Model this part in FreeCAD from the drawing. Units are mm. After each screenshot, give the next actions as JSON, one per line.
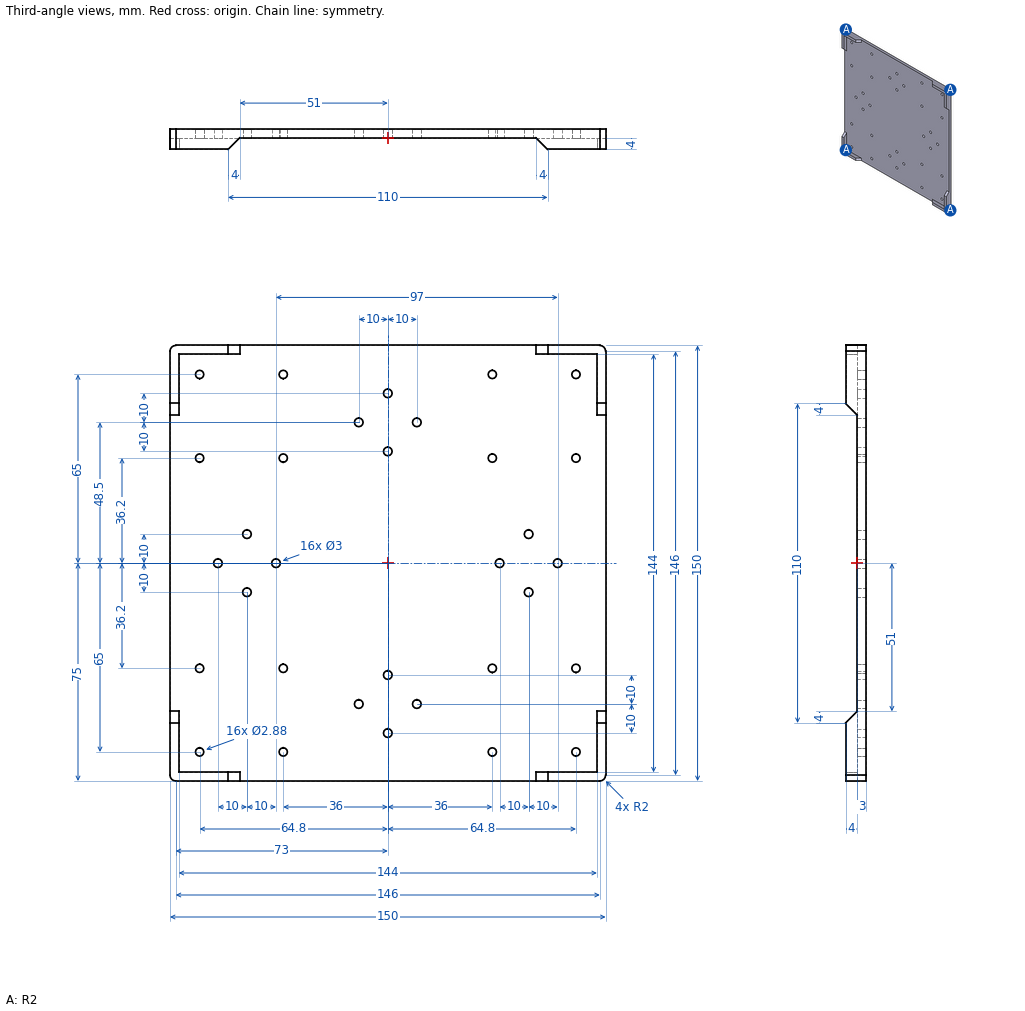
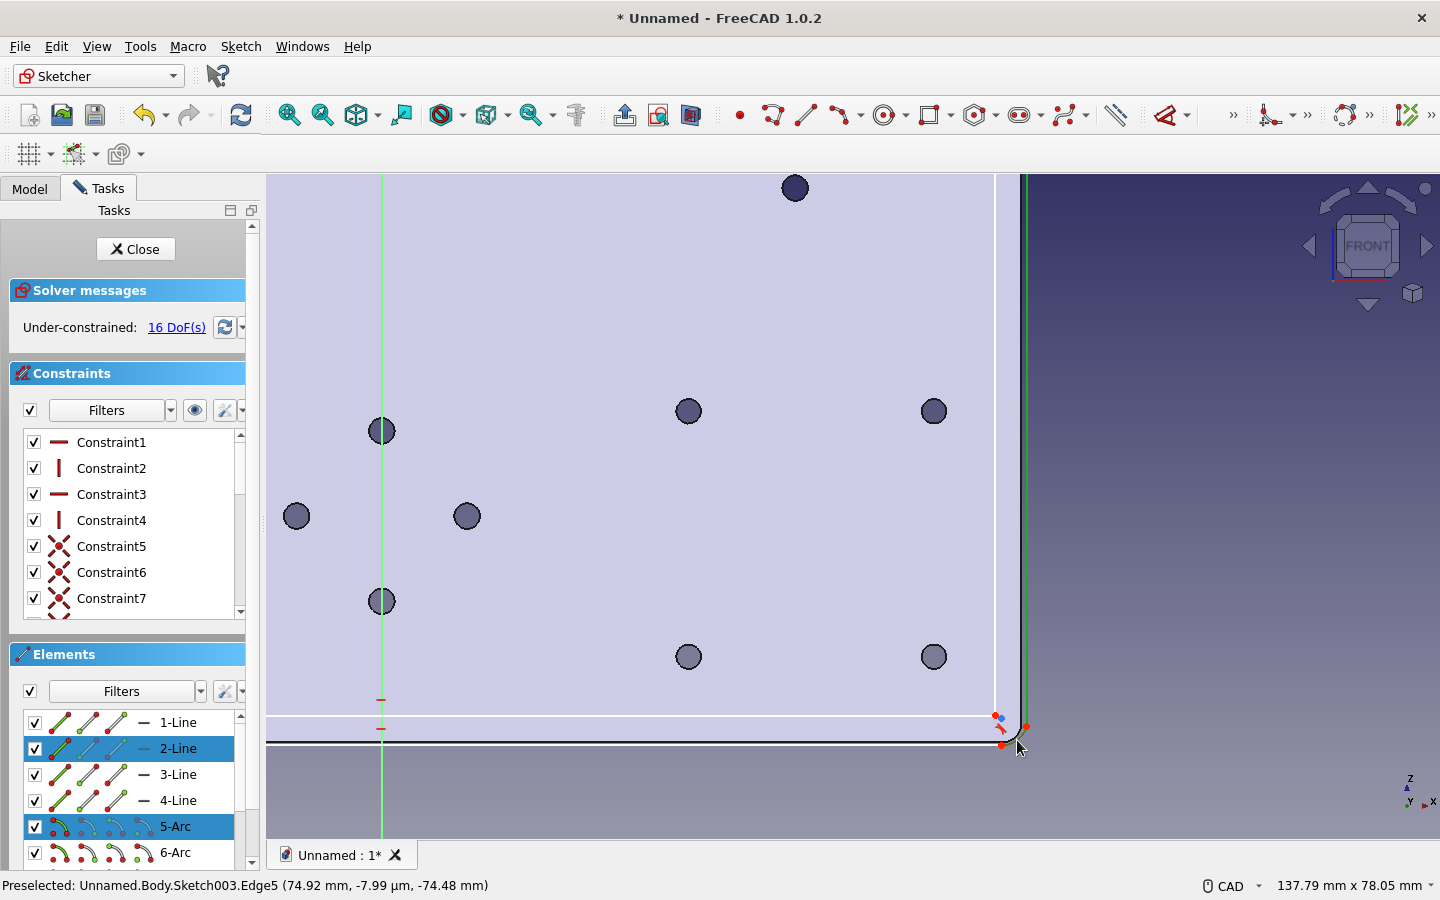
{"action": "key", "text": "t"}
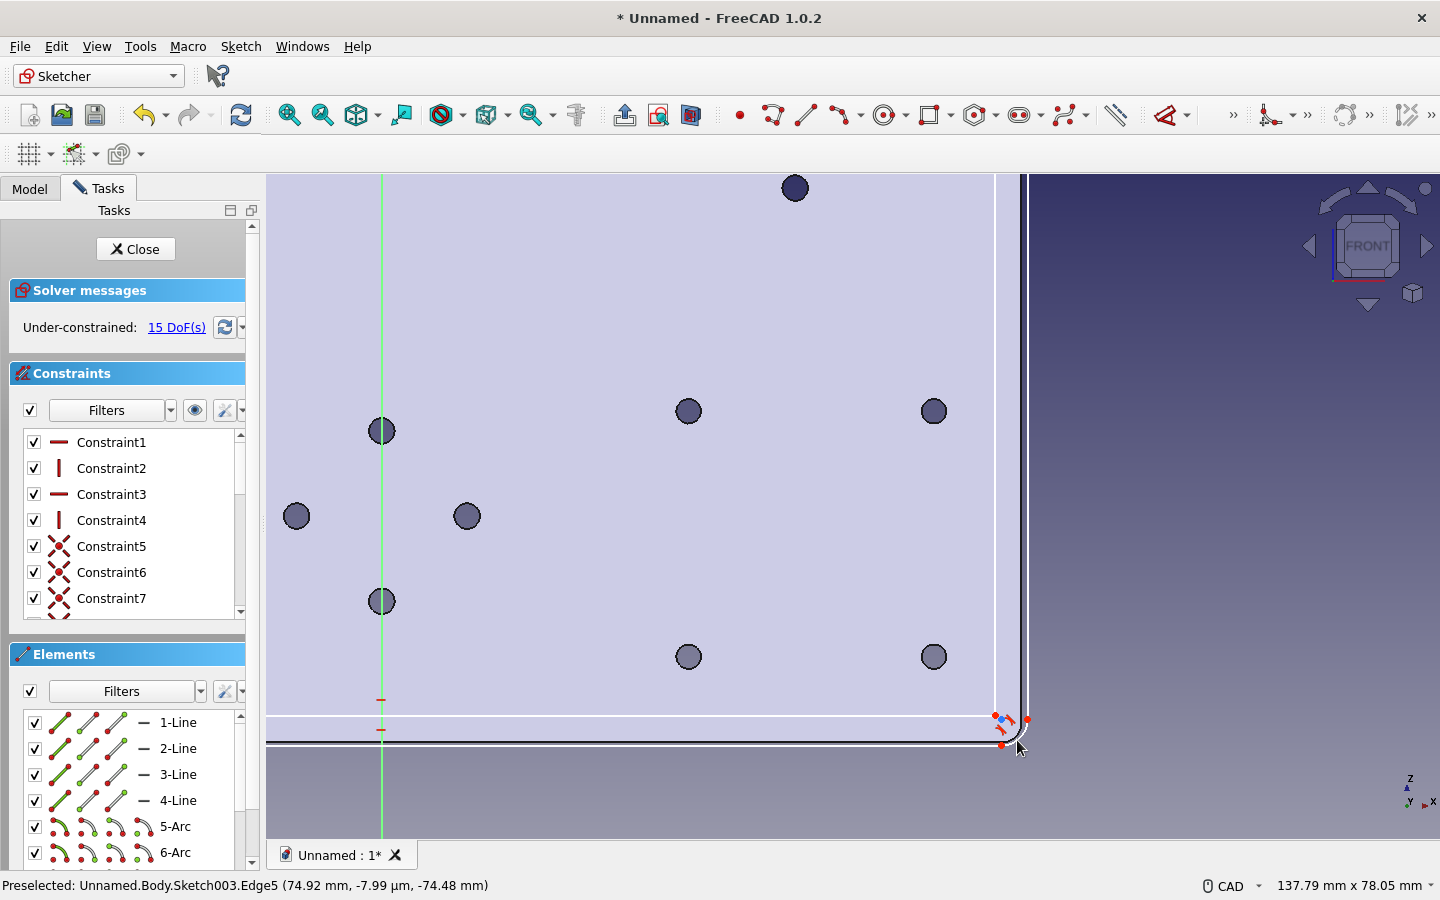
{"action": "left_click", "coordinate": [1028, 349]}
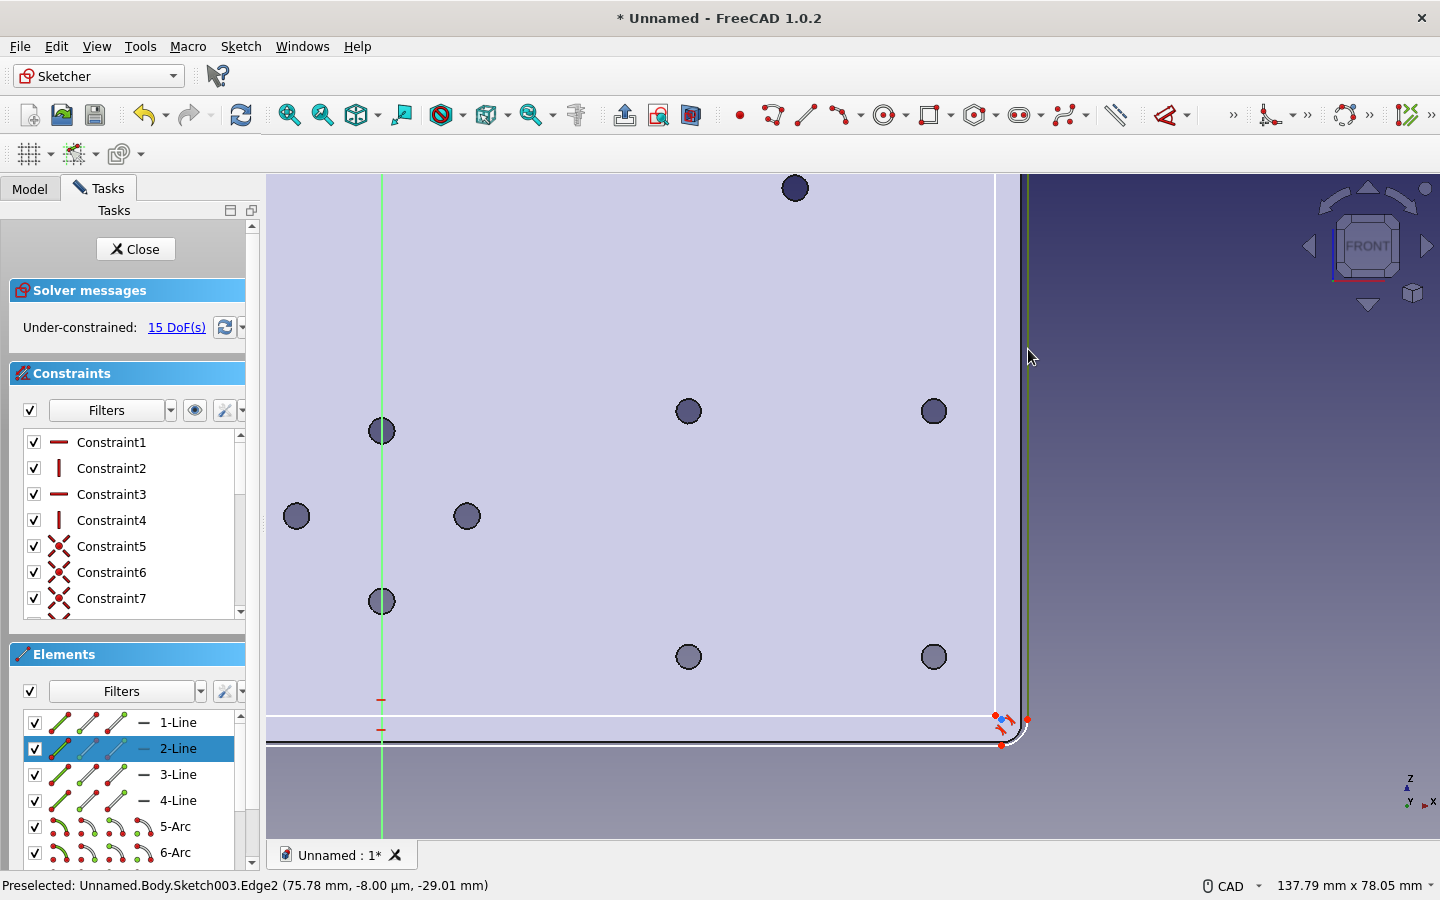
{"action": "scroll", "coordinate": [1019, 741], "scroll_direction": "down", "scroll_amount": 5}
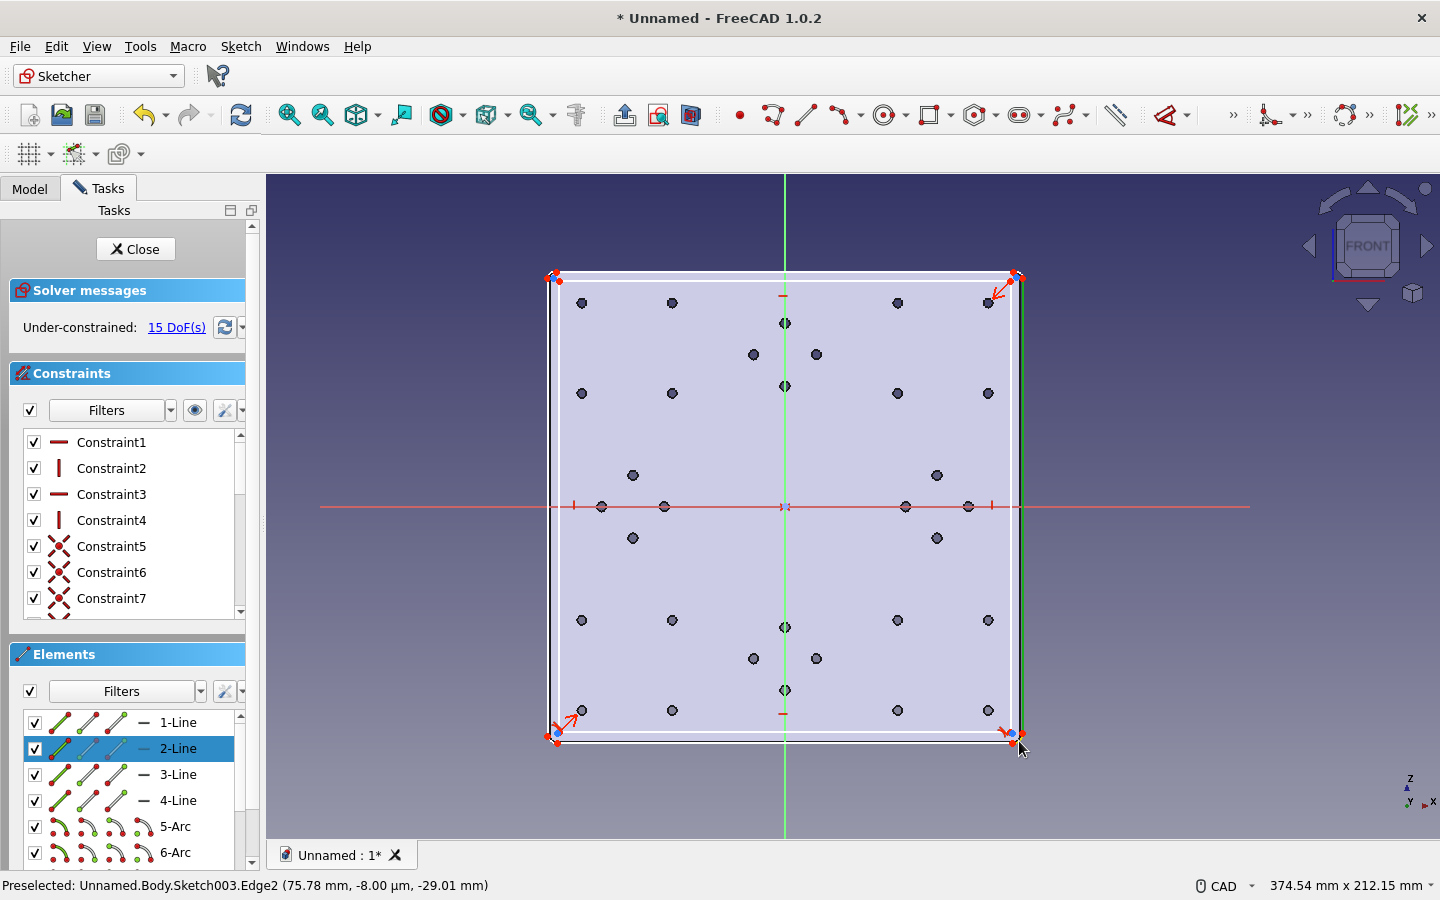
{"action": "scroll", "coordinate": [1022, 275], "scroll_direction": "up", "scroll_amount": 7}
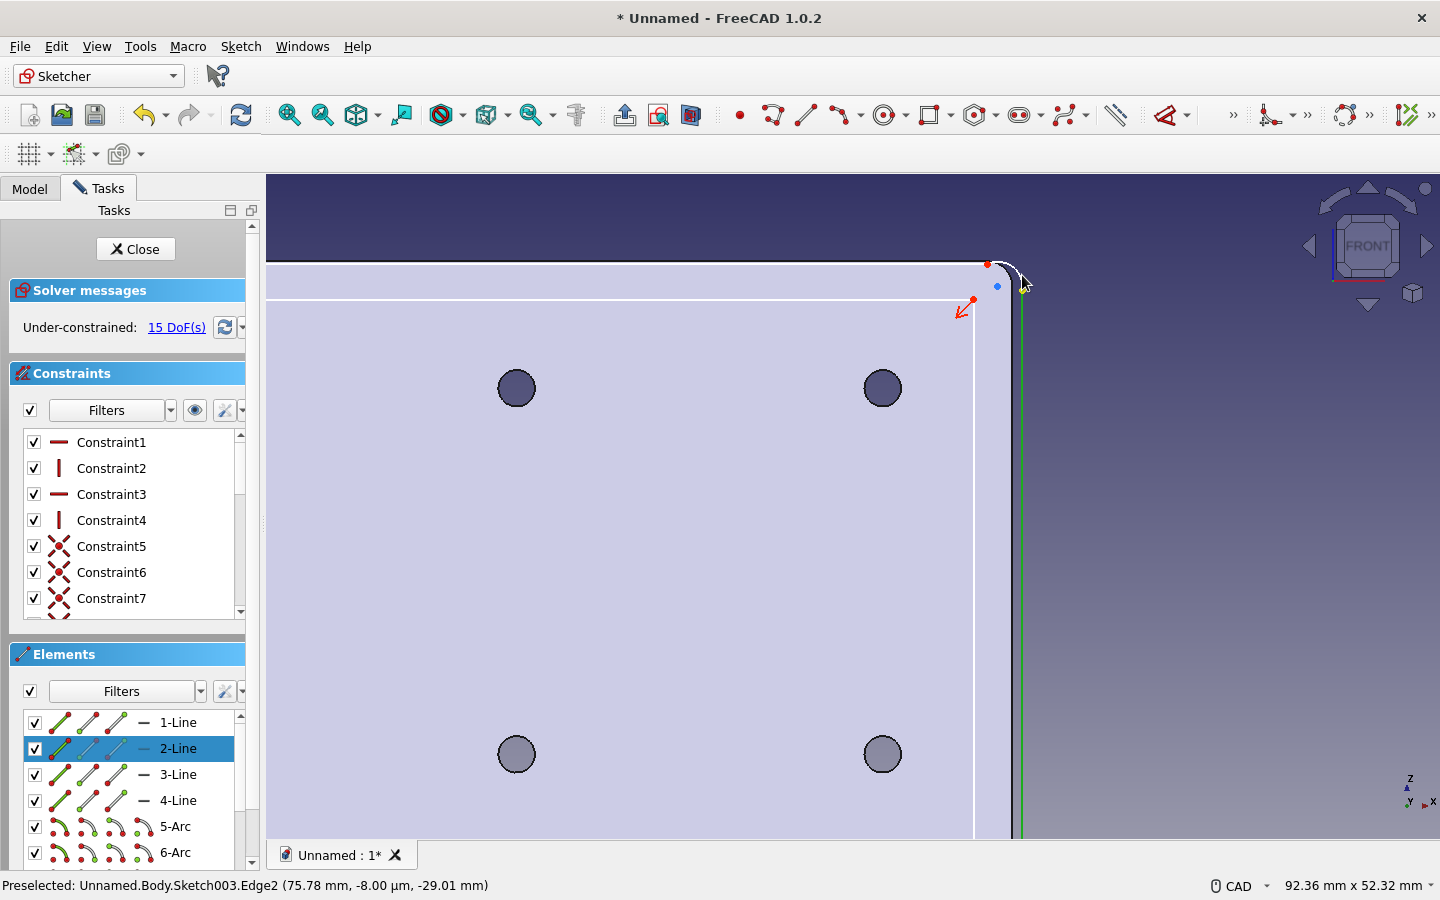
{"action": "left_click", "coordinate": [1019, 275]}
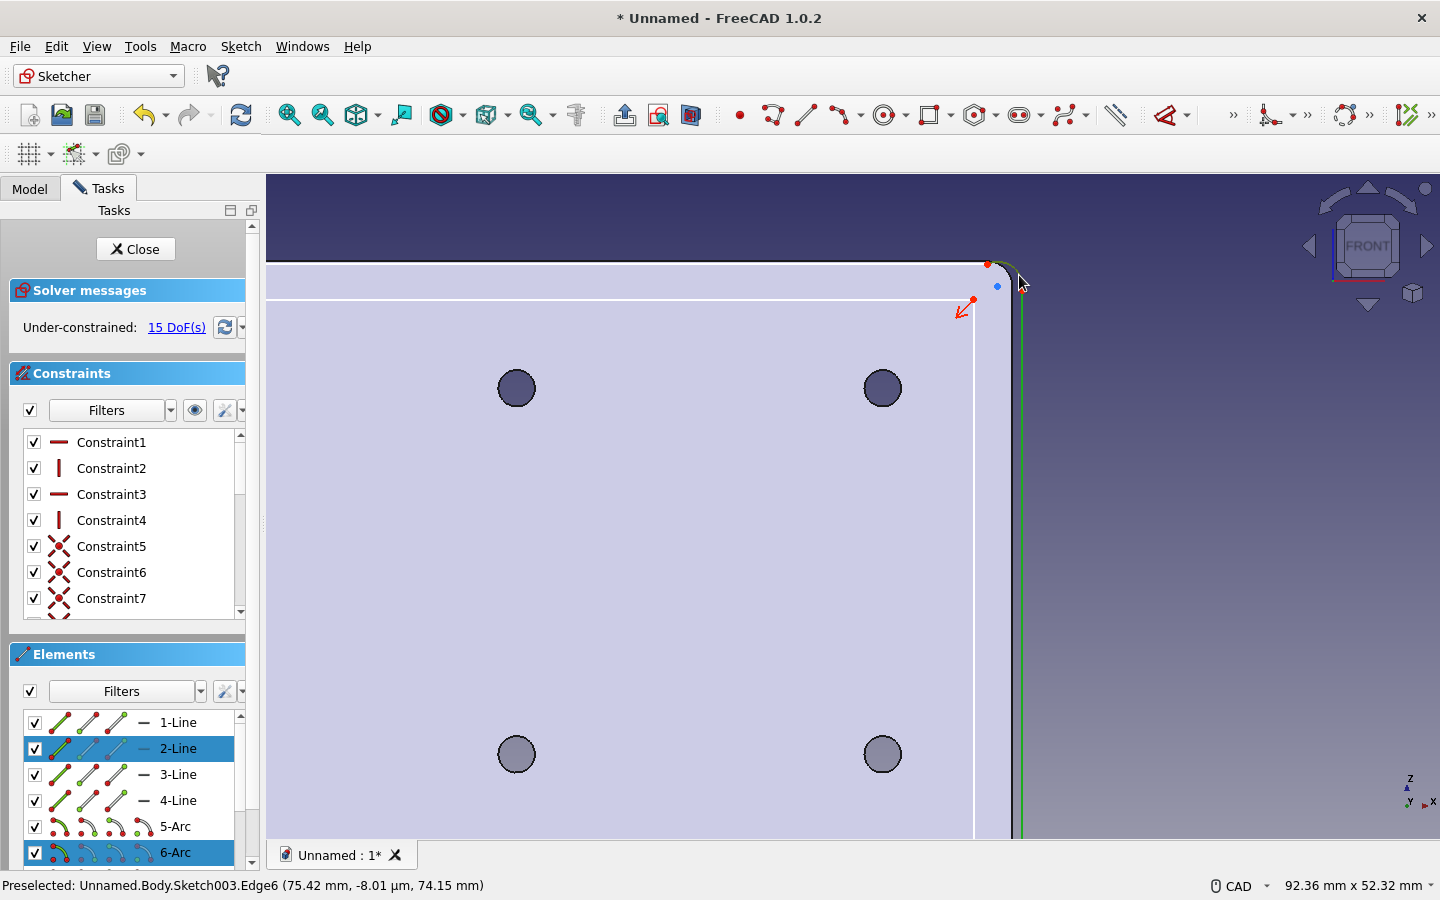
{"action": "key", "text": "t"}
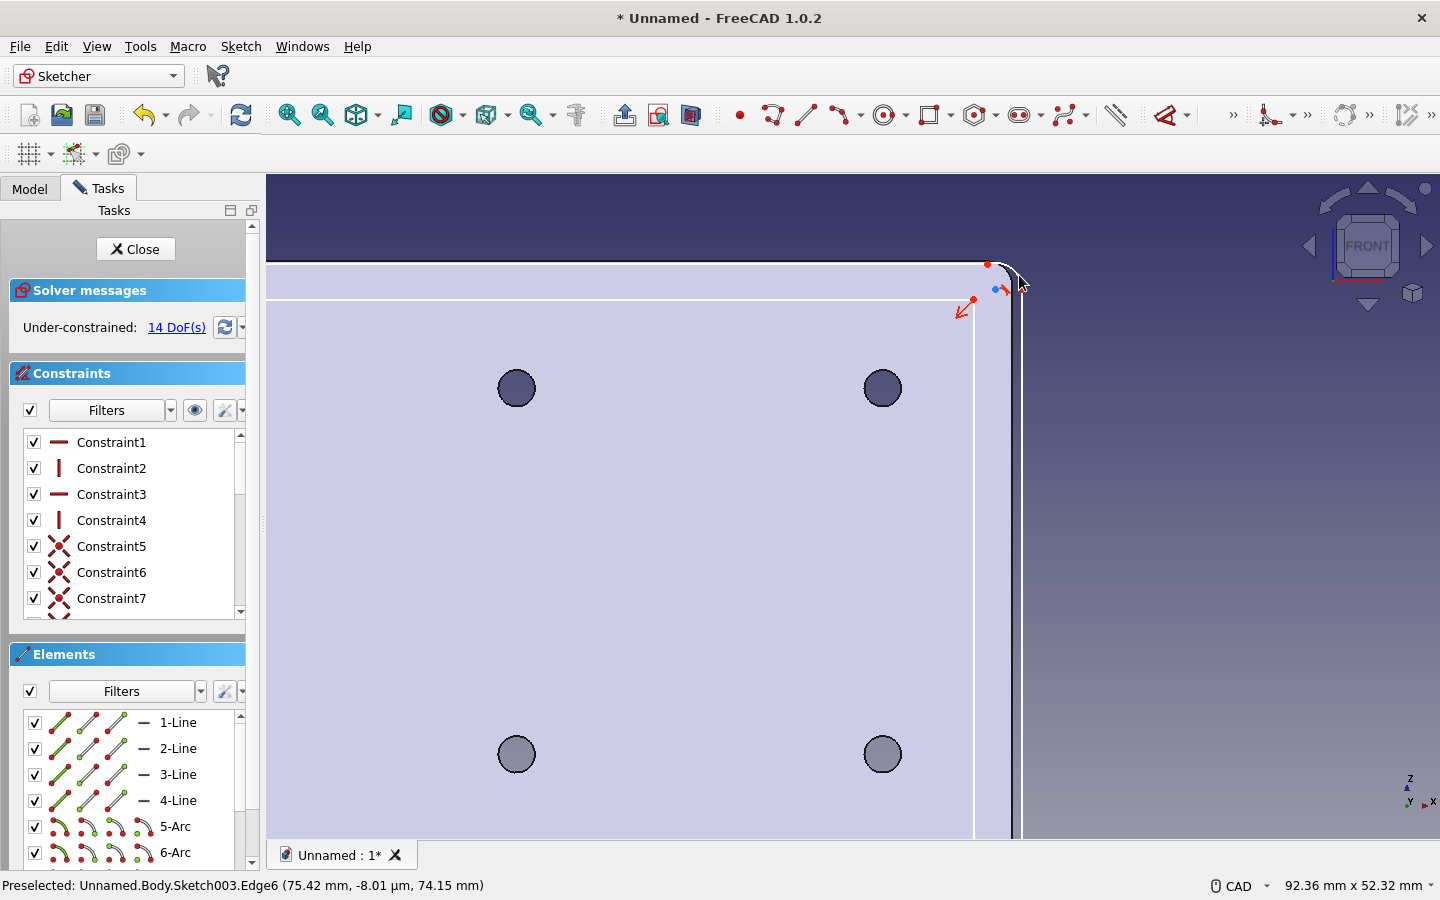
{"action": "left_click", "coordinate": [431, 264]}